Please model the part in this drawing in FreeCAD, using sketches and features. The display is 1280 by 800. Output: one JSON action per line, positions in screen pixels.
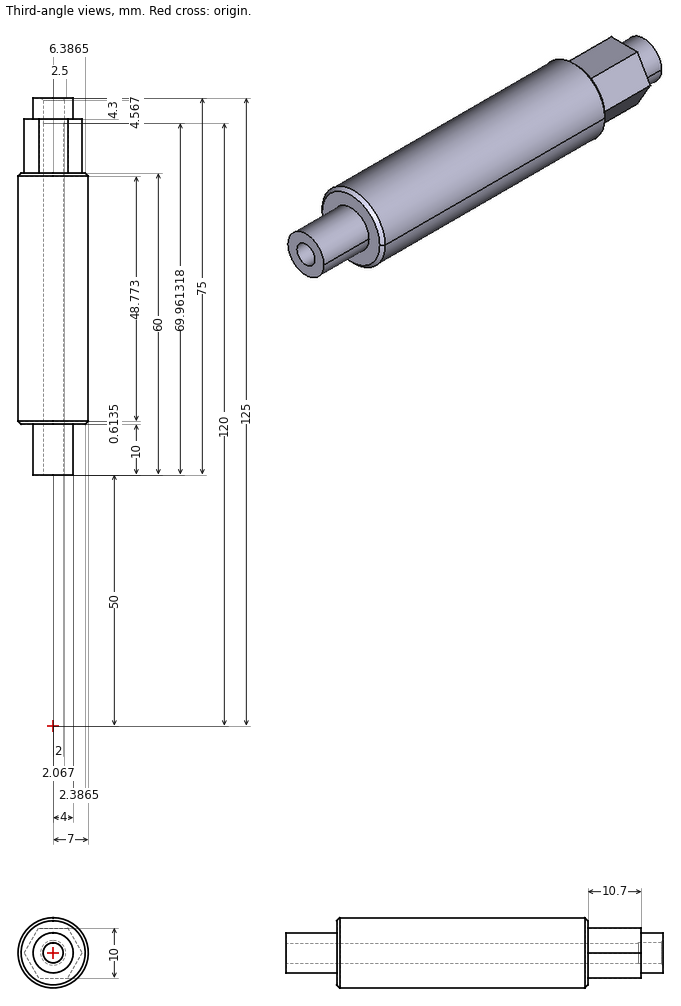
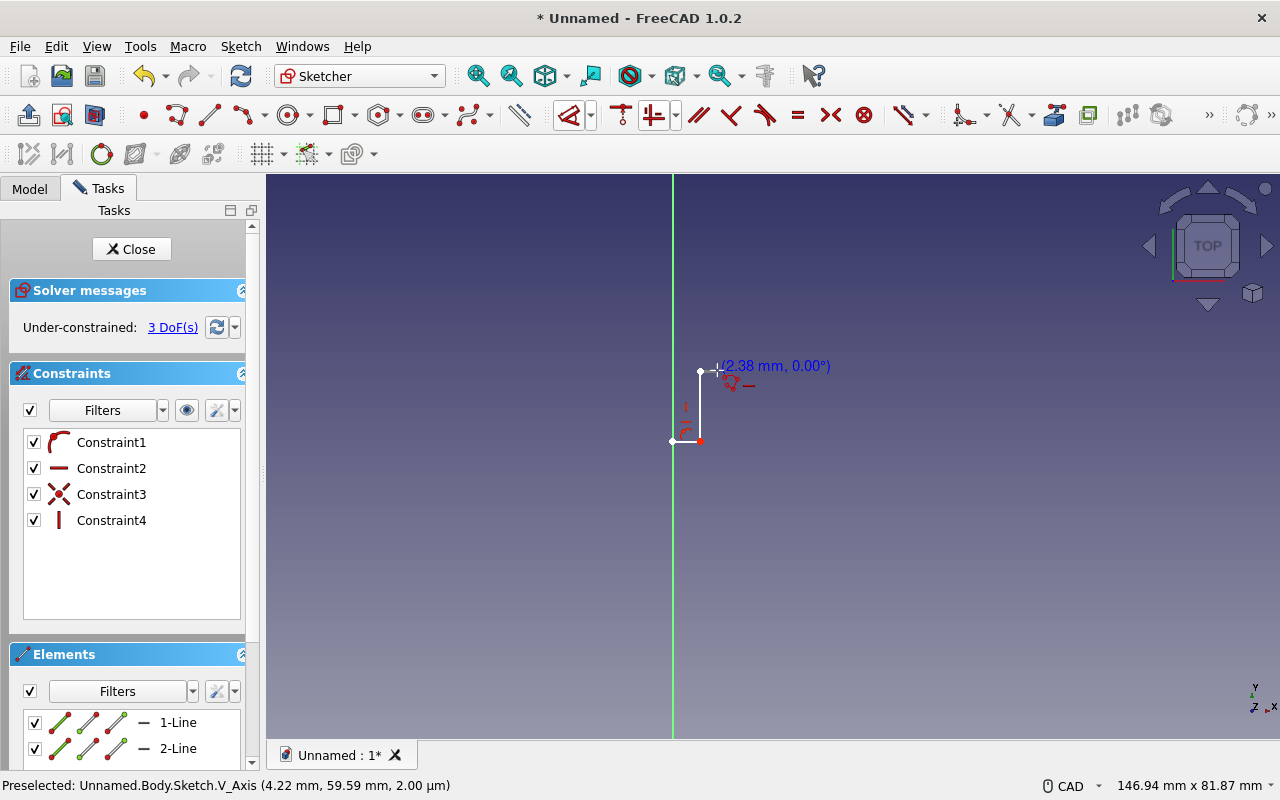
{"action": "left_click", "coordinate": [717, 370]}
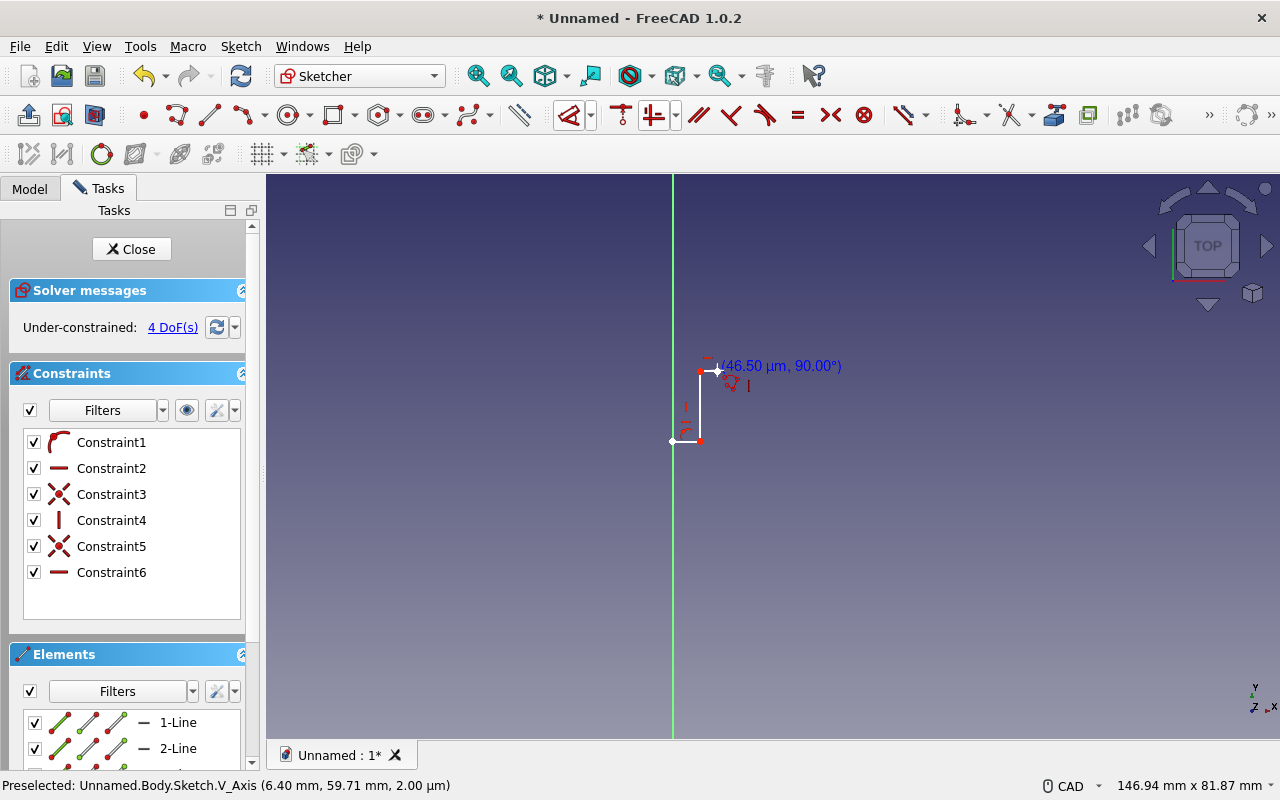
{"action": "scroll", "coordinate": [721, 366], "scroll_direction": "up", "scroll_amount": 5}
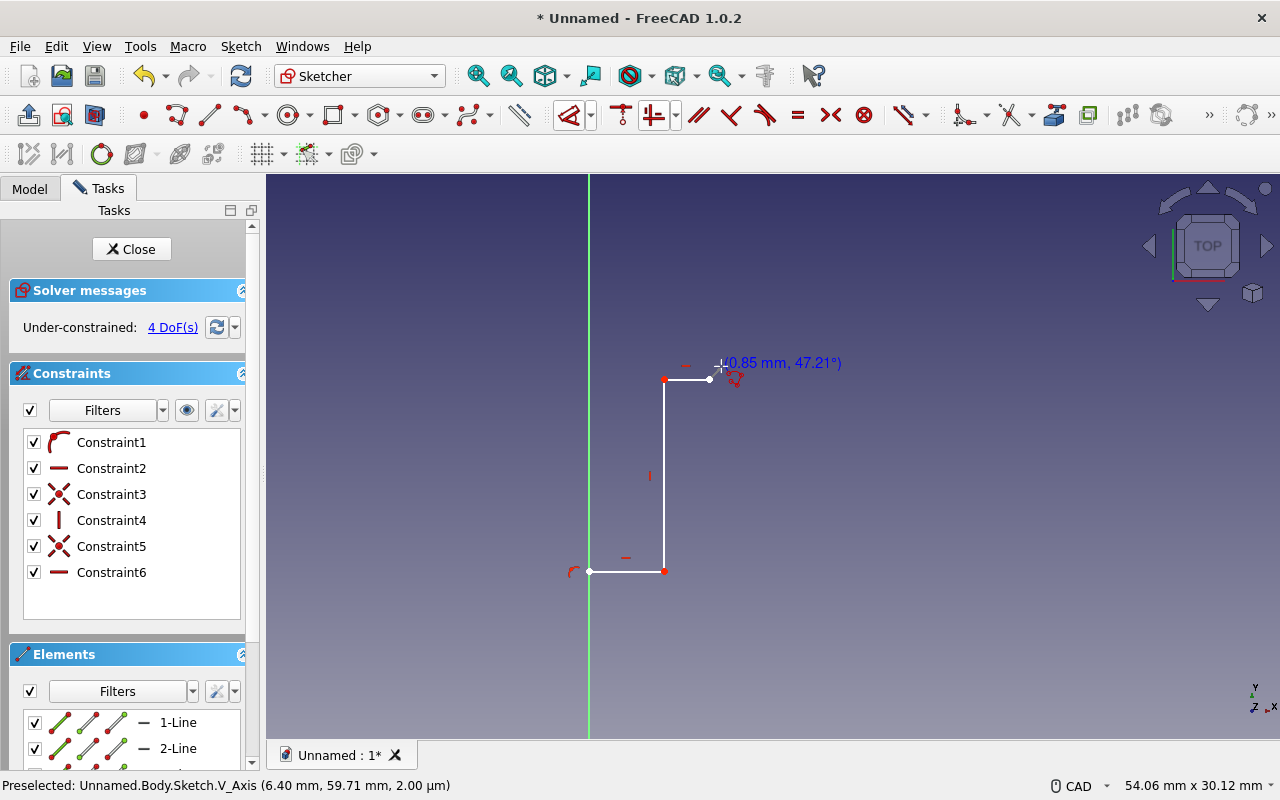
{"action": "left_click", "coordinate": [720, 365]}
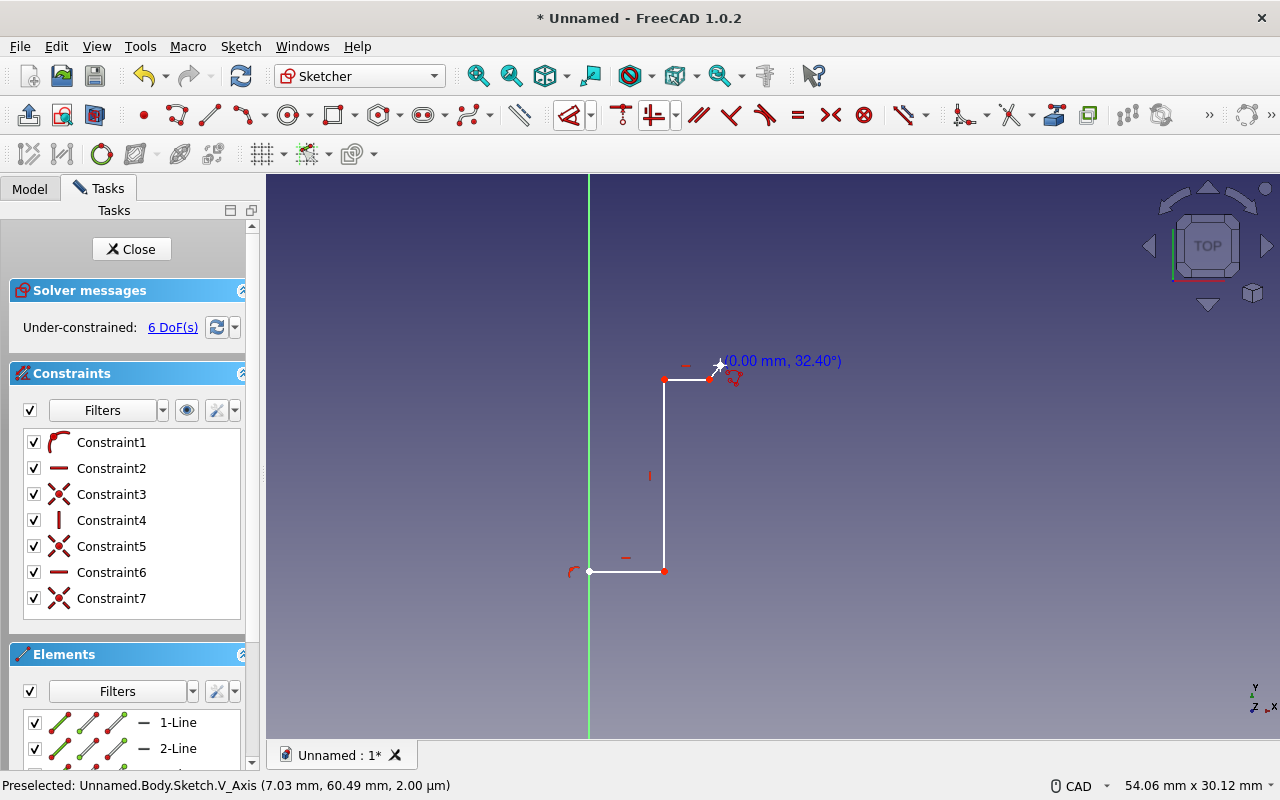
{"action": "scroll", "coordinate": [714, 454], "scroll_direction": "down", "scroll_amount": 9}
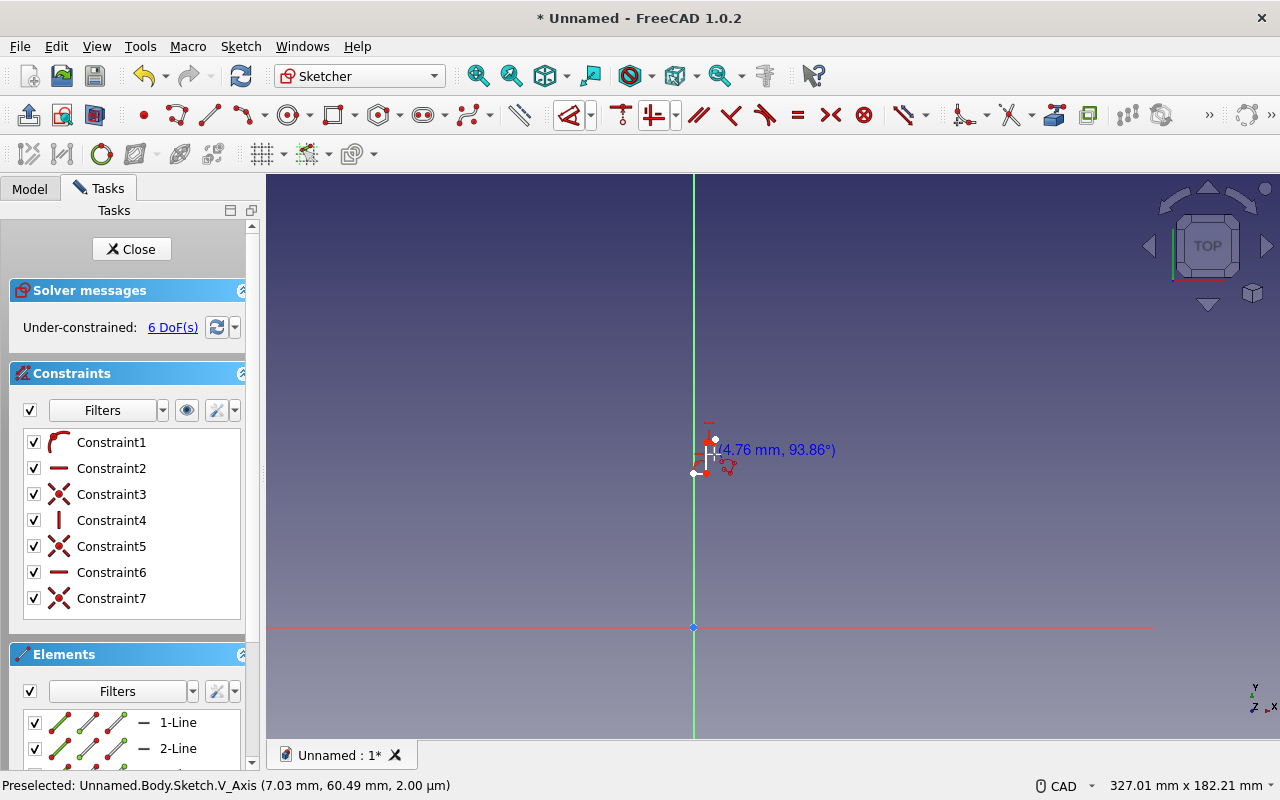
{"action": "left_click", "coordinate": [715, 288]}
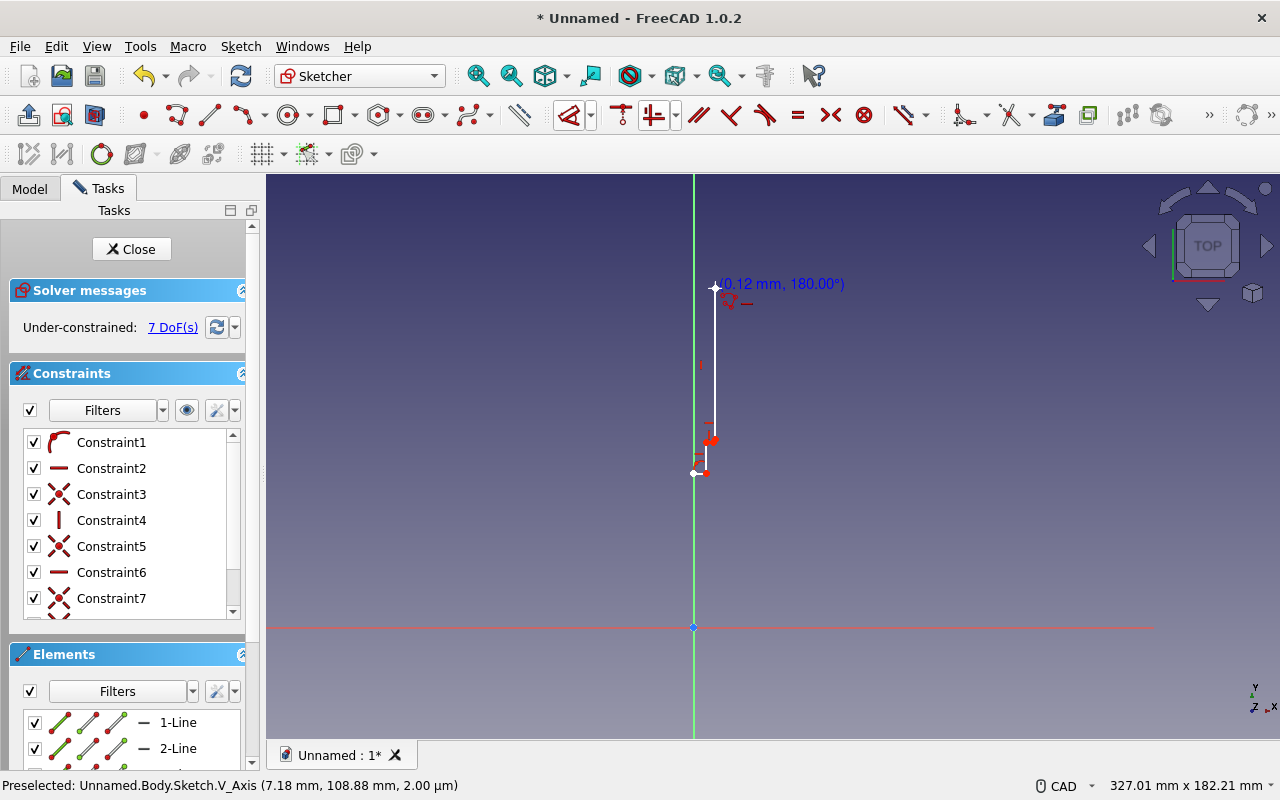
{"action": "scroll", "coordinate": [714, 287], "scroll_direction": "up", "scroll_amount": 9}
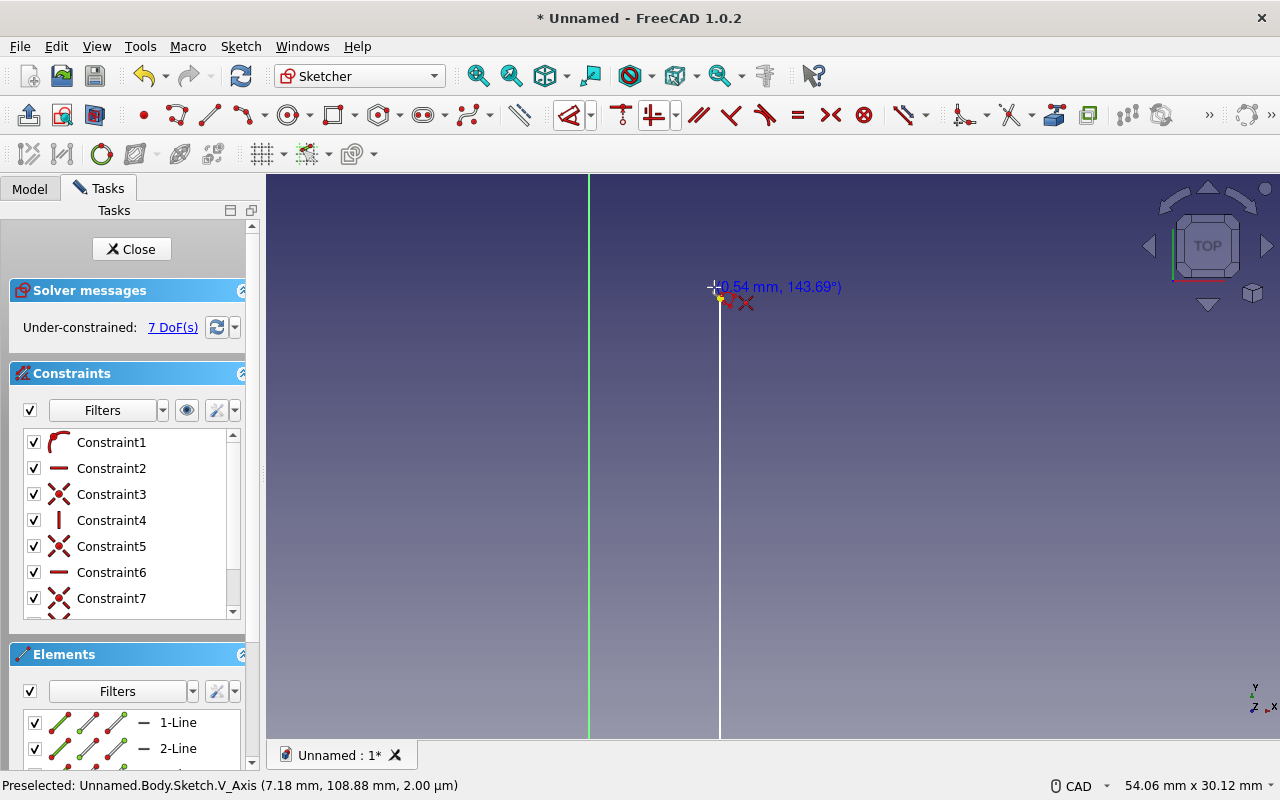
{"action": "left_click", "coordinate": [709, 283]}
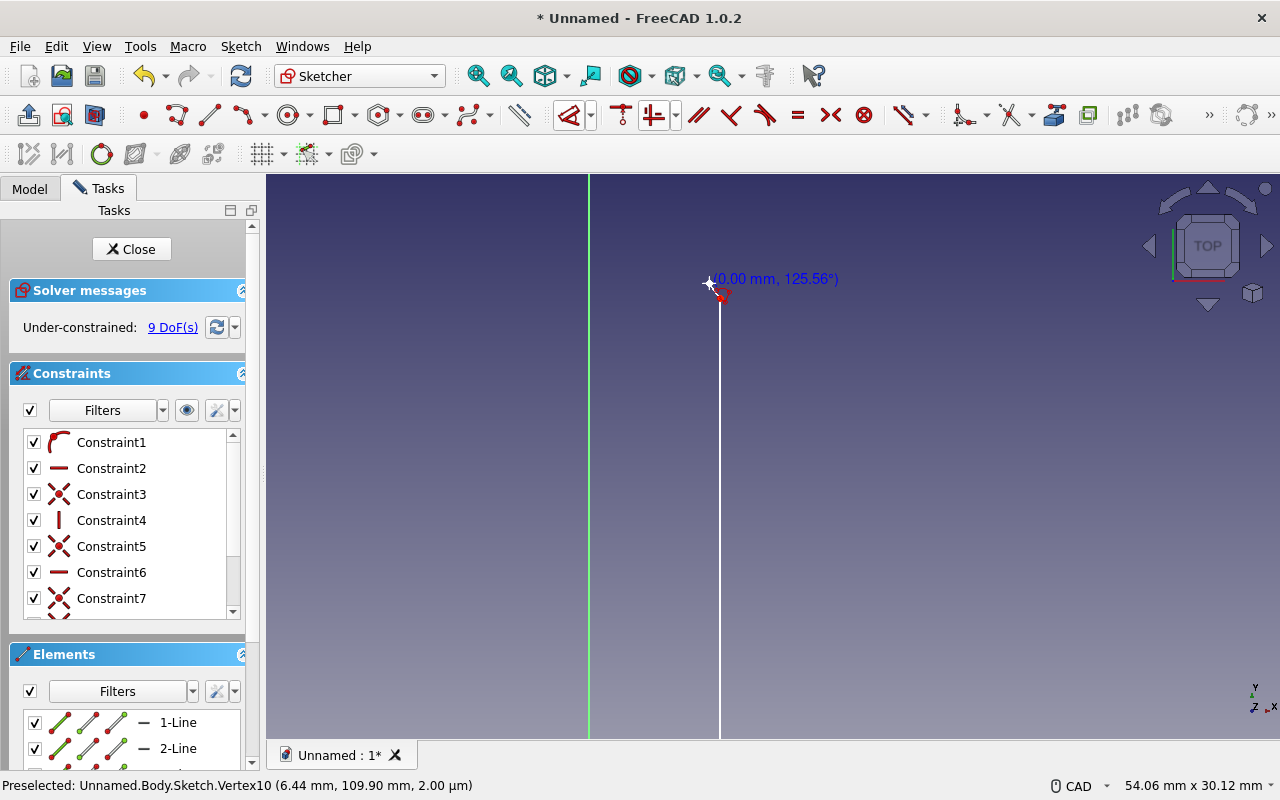
{"action": "scroll", "coordinate": [714, 287], "scroll_direction": "down", "scroll_amount": 9}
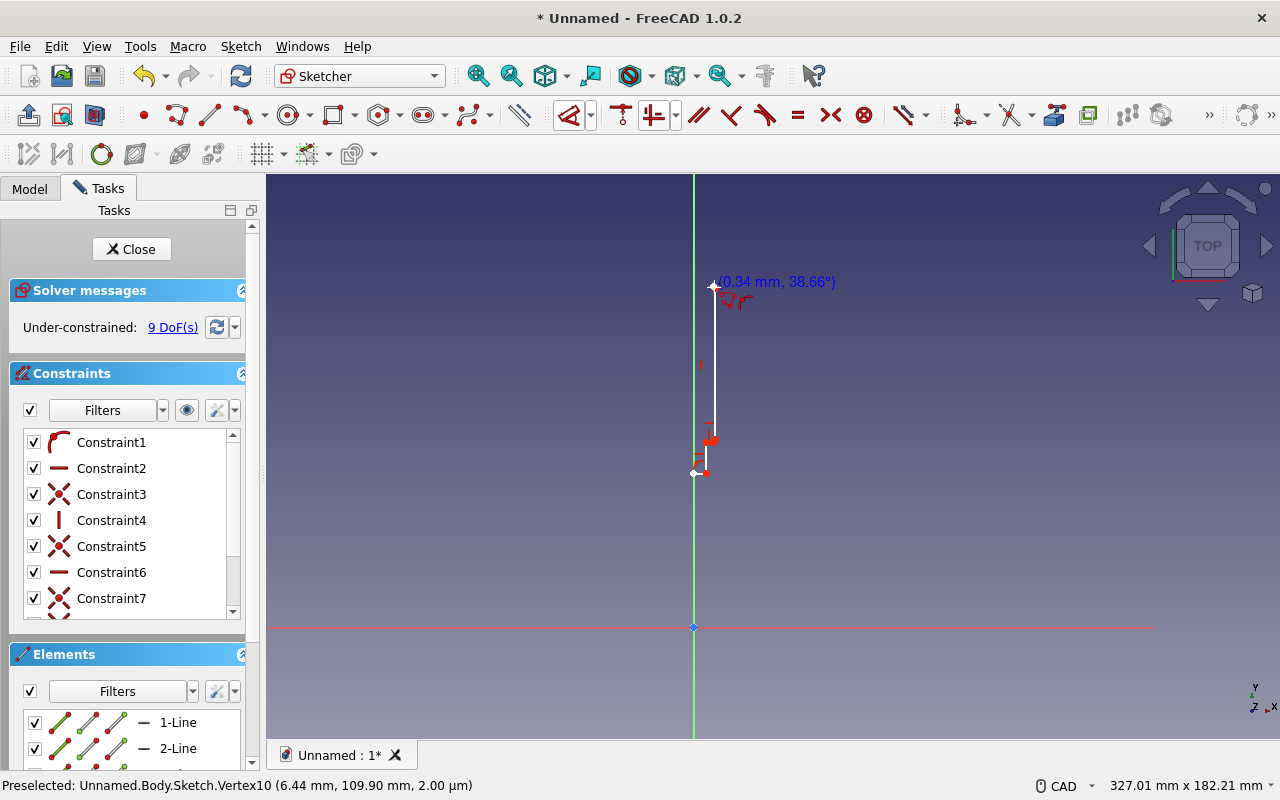
{"action": "left_click", "coordinate": [703, 287]}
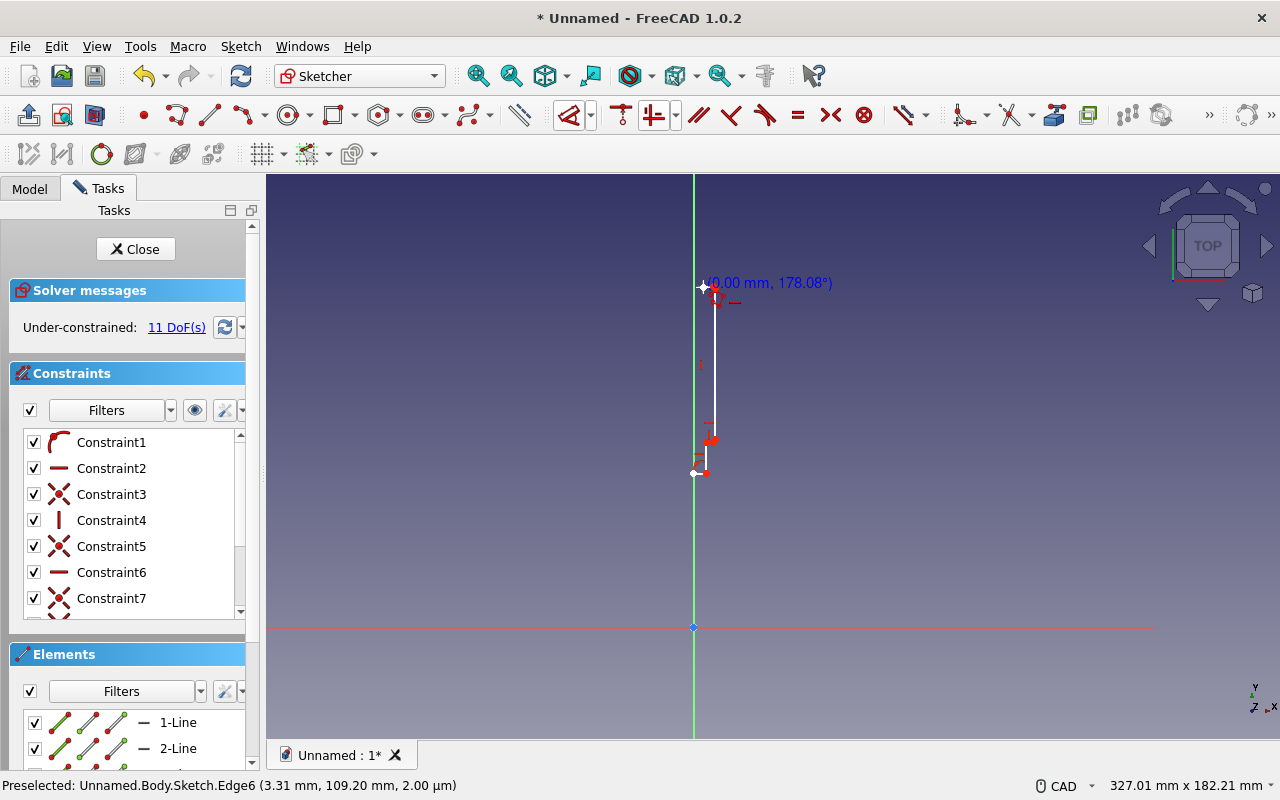
{"action": "scroll", "coordinate": [694, 473], "scroll_direction": "up", "scroll_amount": 5}